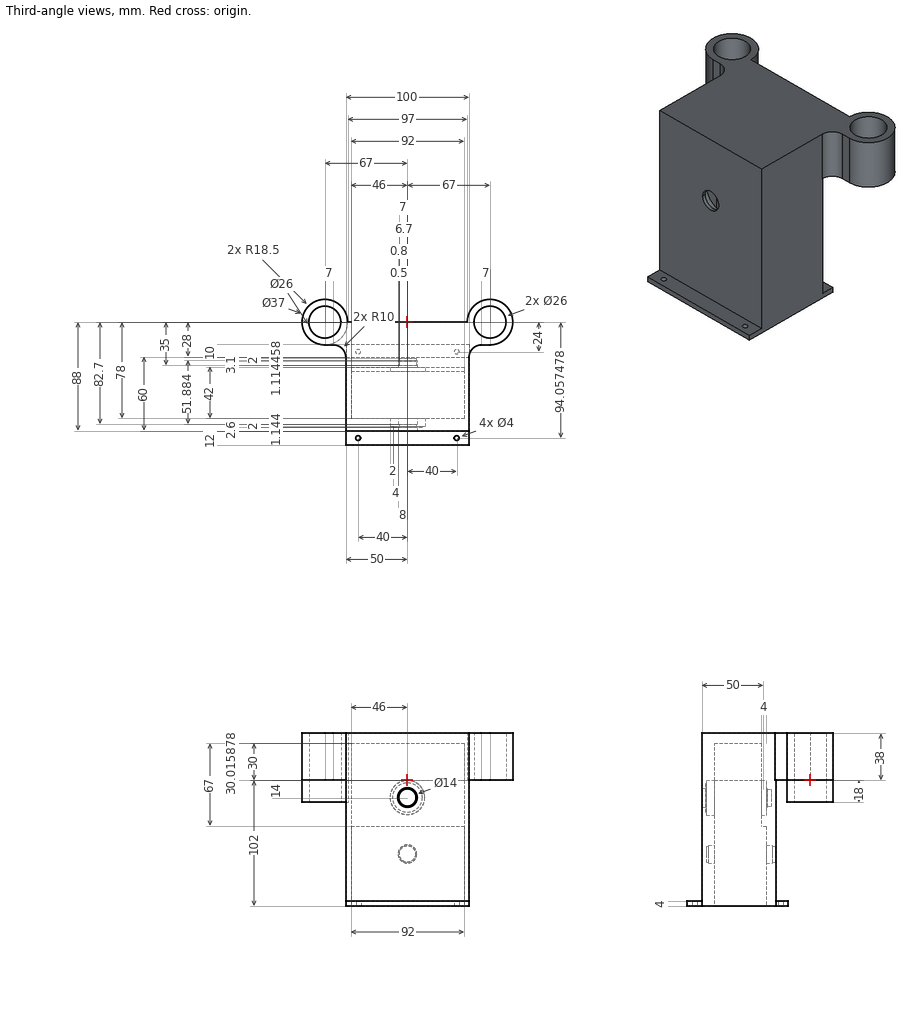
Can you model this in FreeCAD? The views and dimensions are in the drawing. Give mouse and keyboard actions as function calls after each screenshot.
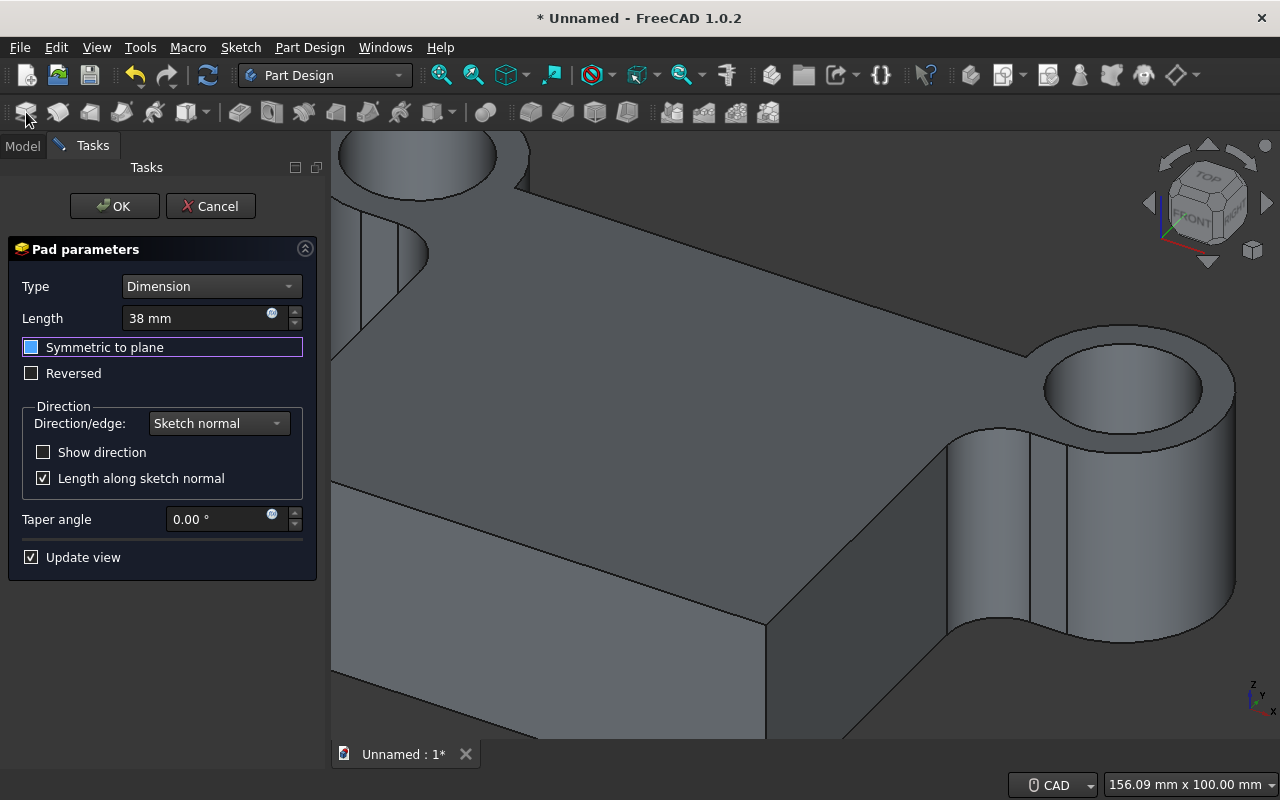
click(115, 206)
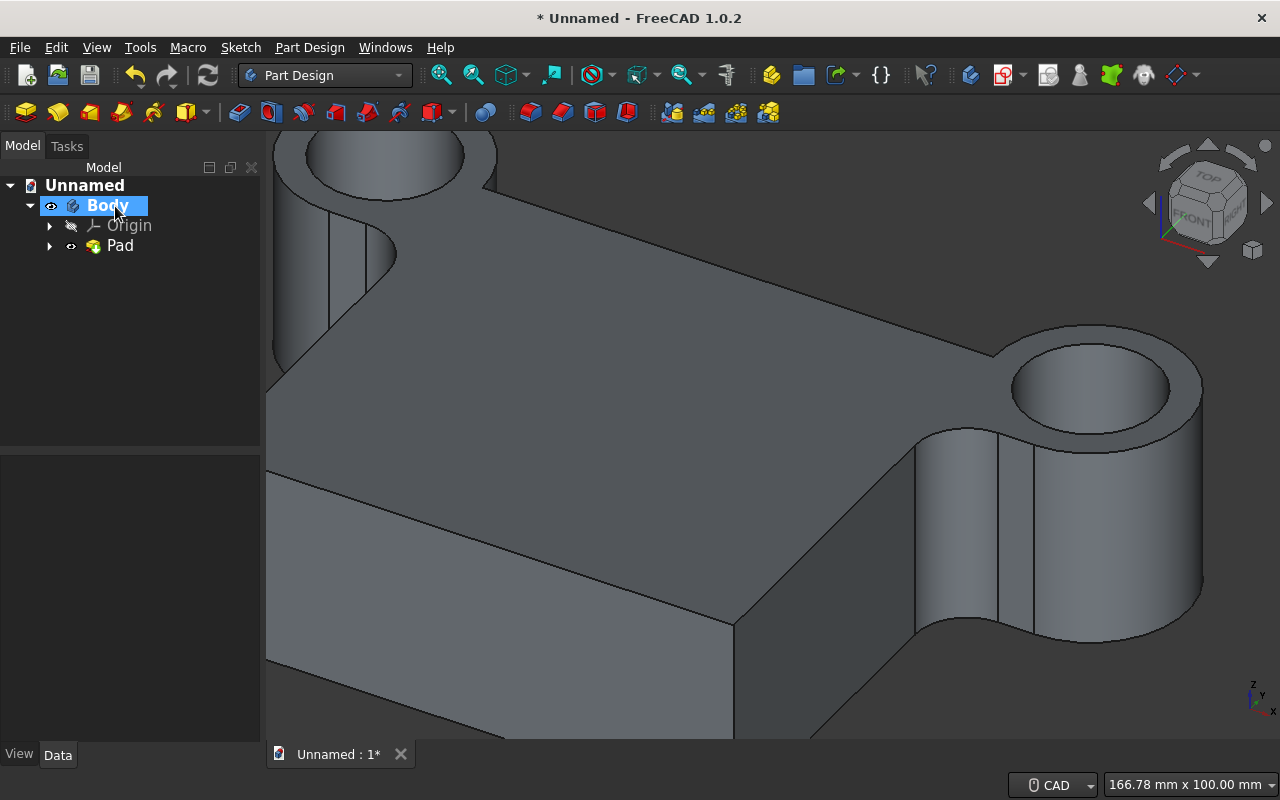
key(v)
key(f)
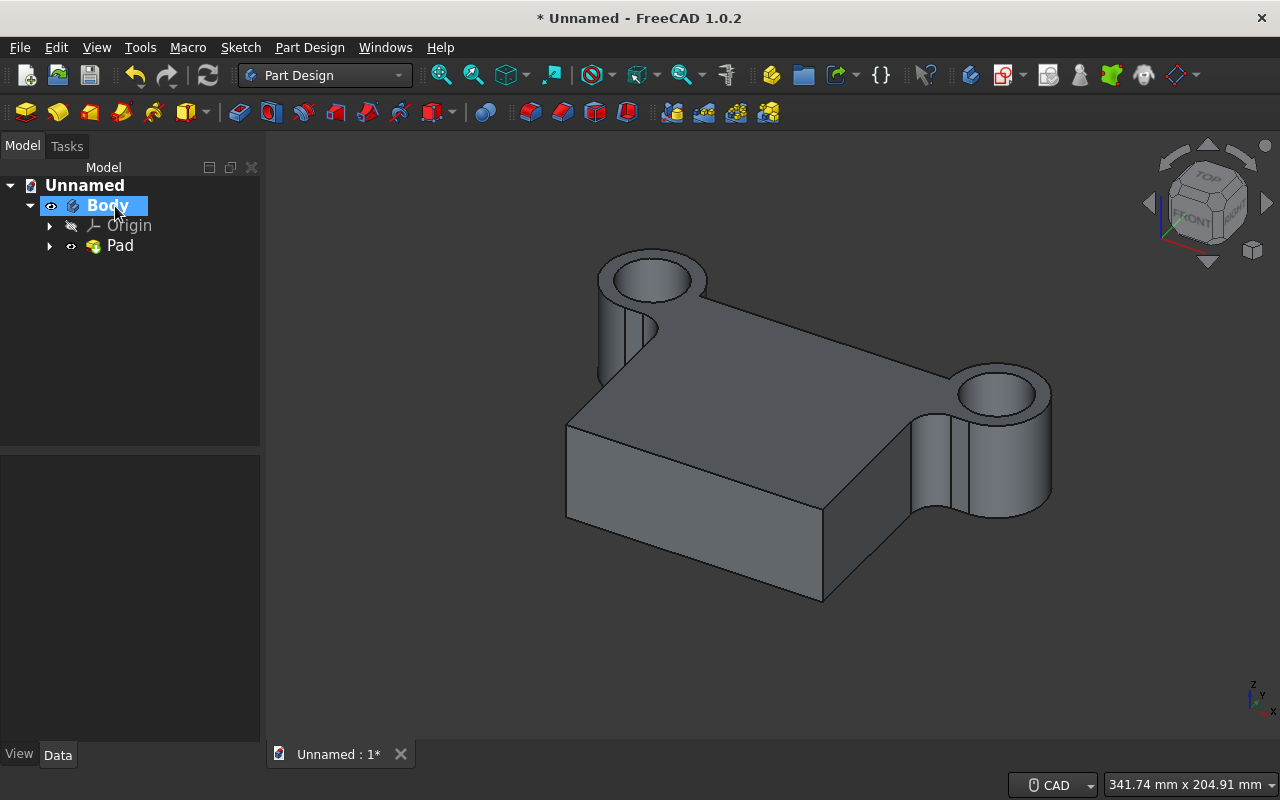
key(5)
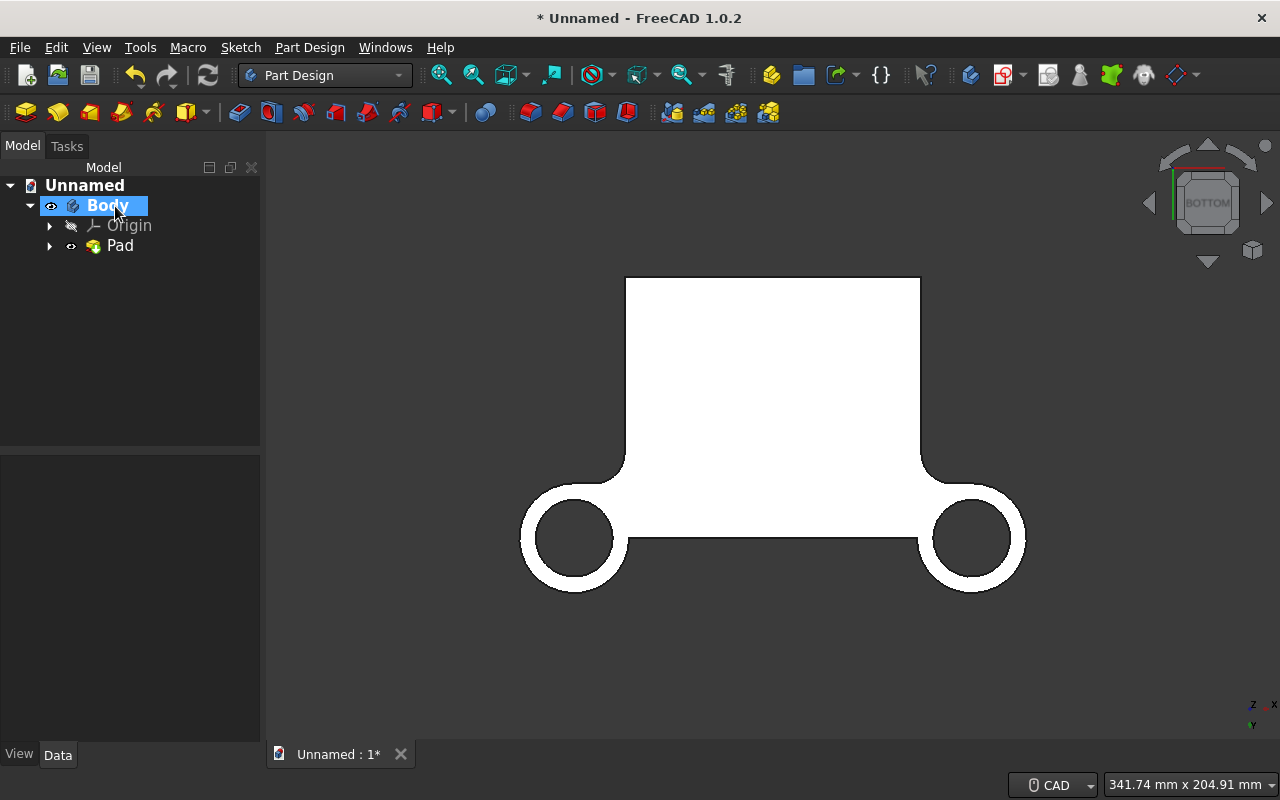
click(773, 389)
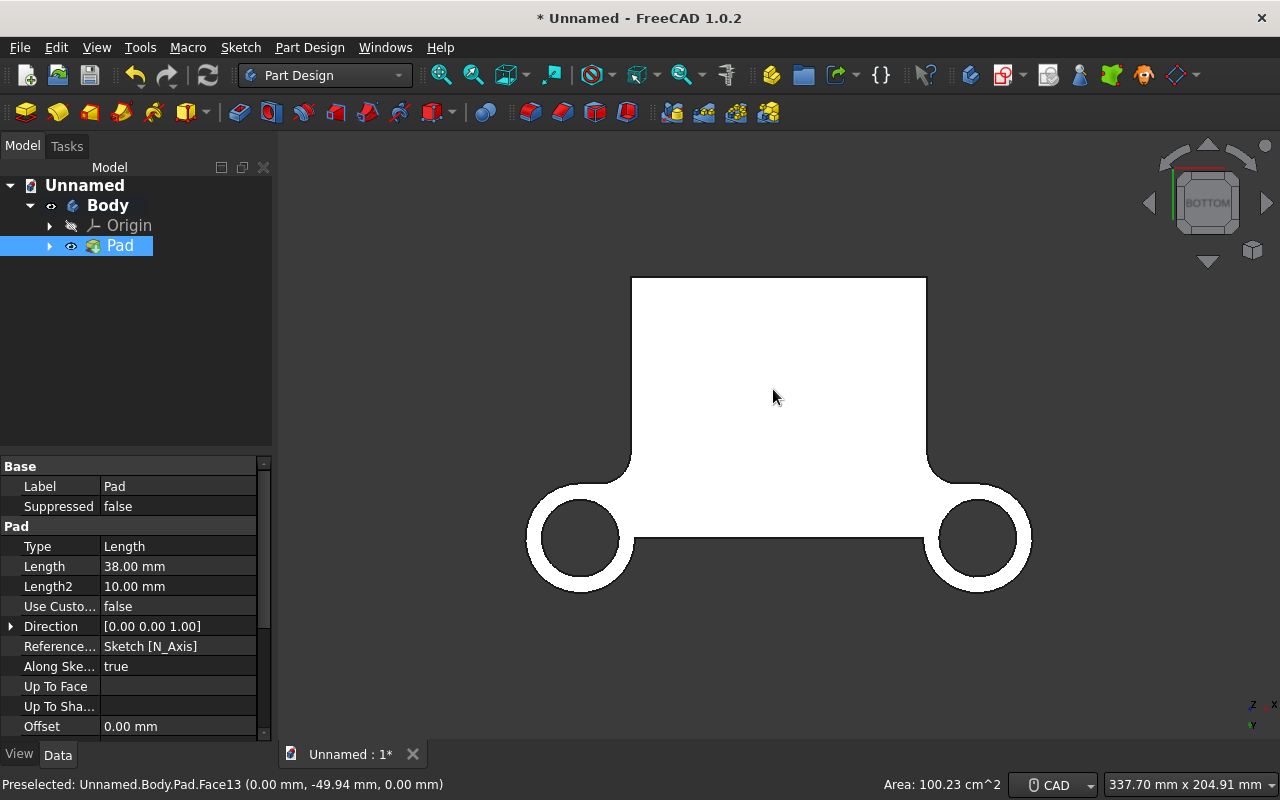
click(1004, 76)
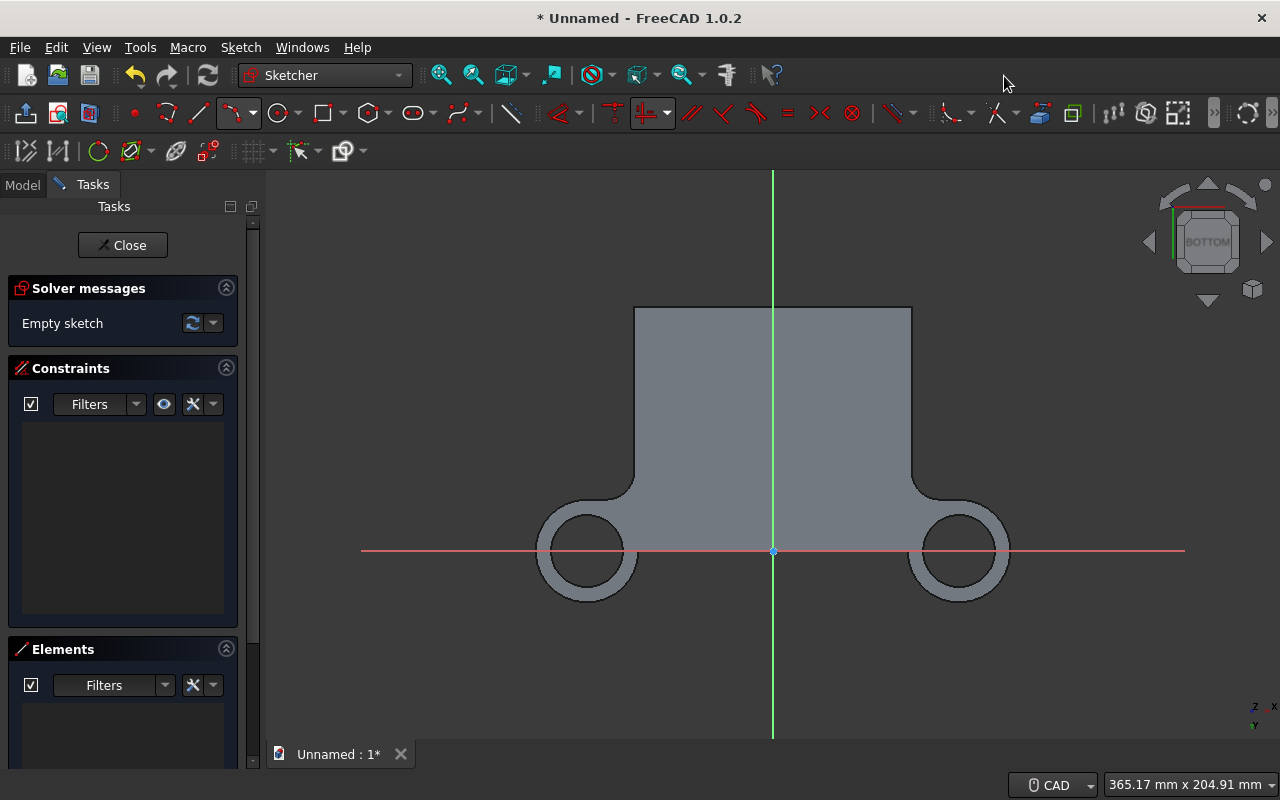
scroll(912, 377, up, 2)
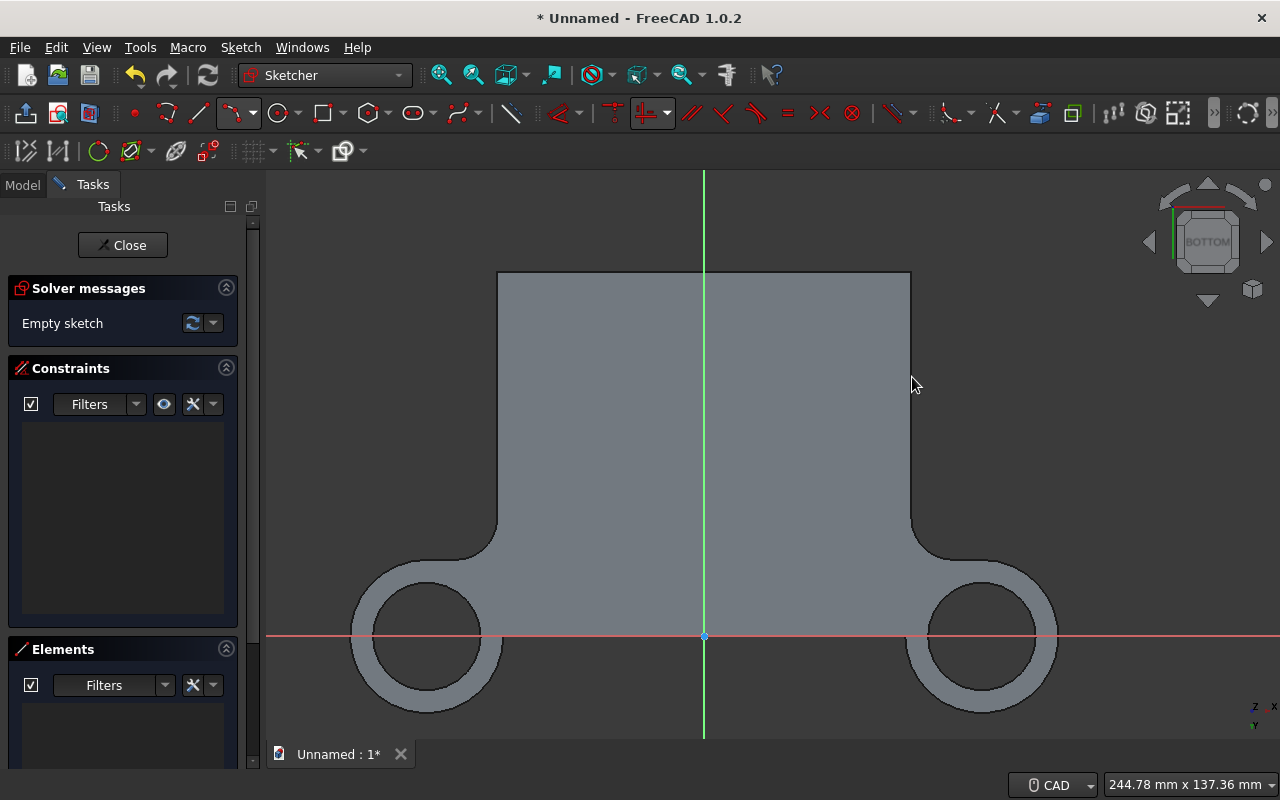
key(g)
key(r)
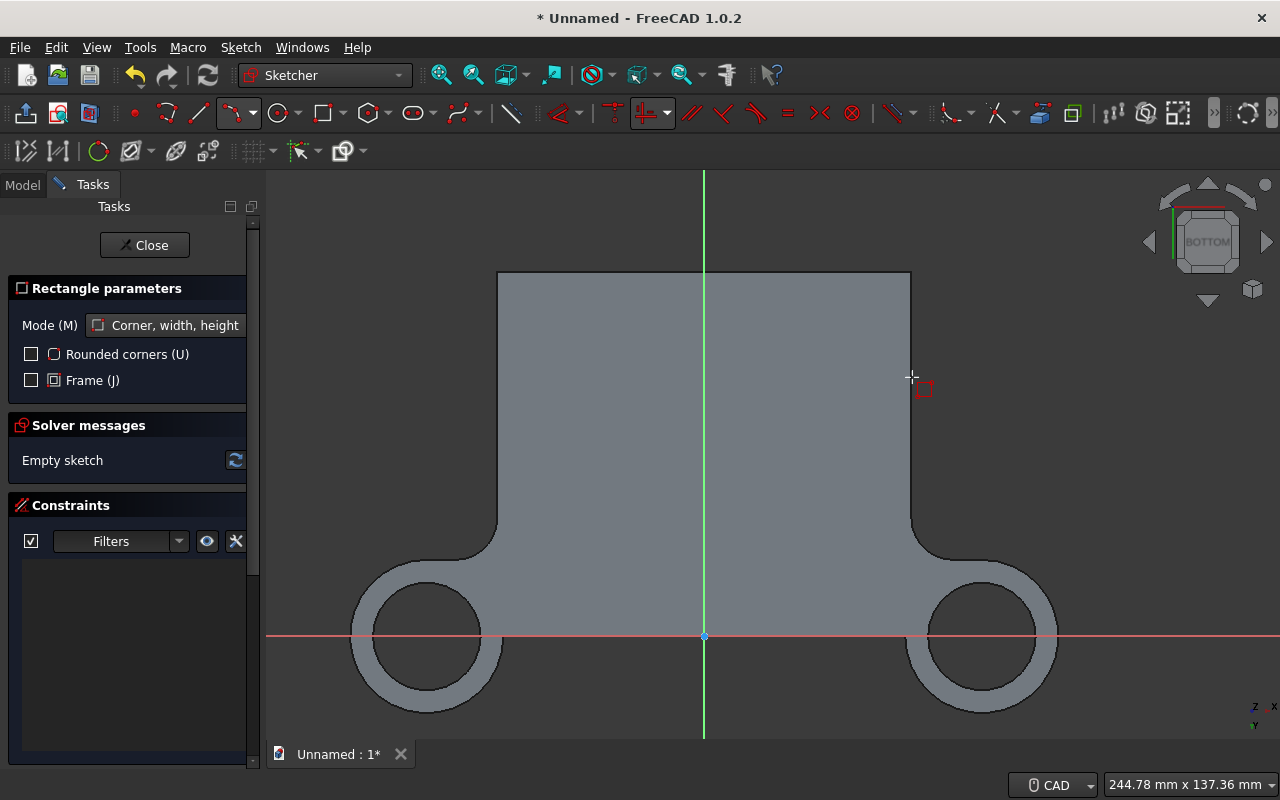
click(497, 272)
click(911, 520)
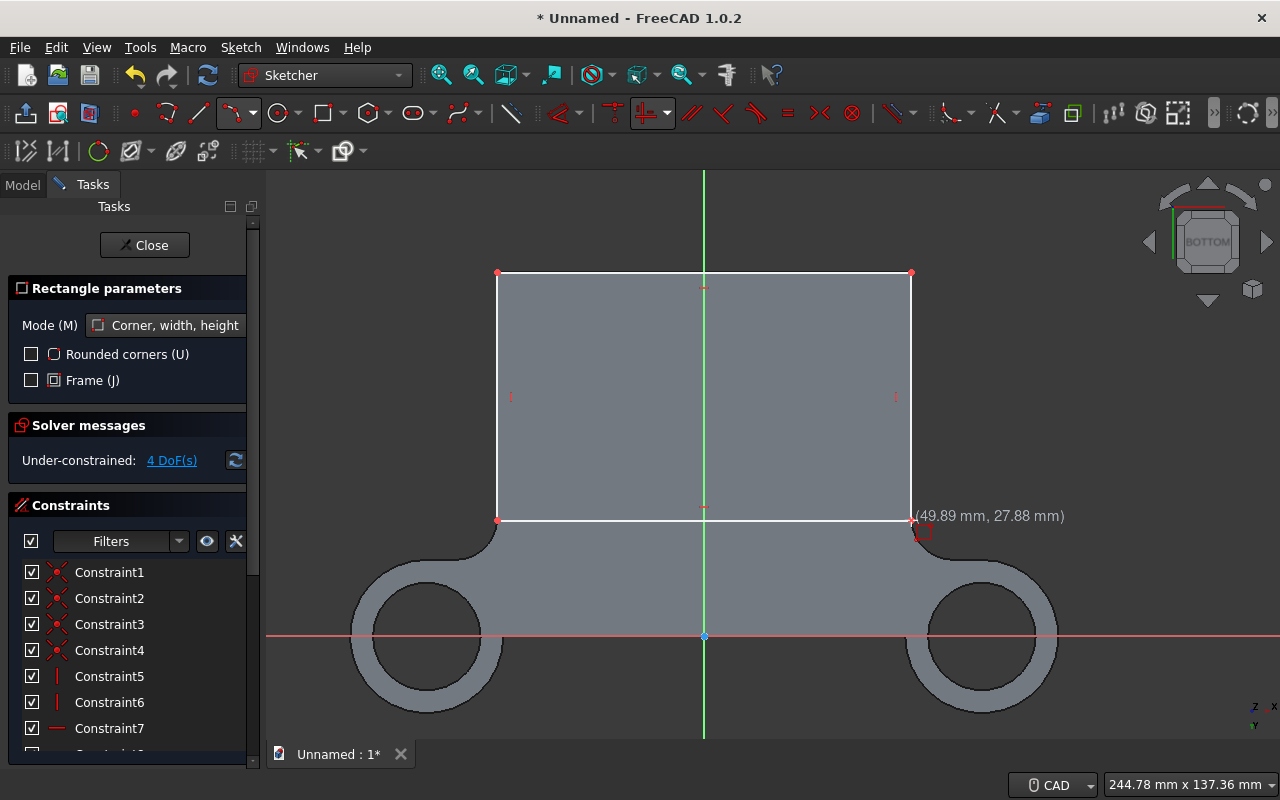
click(514, 313)
click(895, 487)
key(Escape)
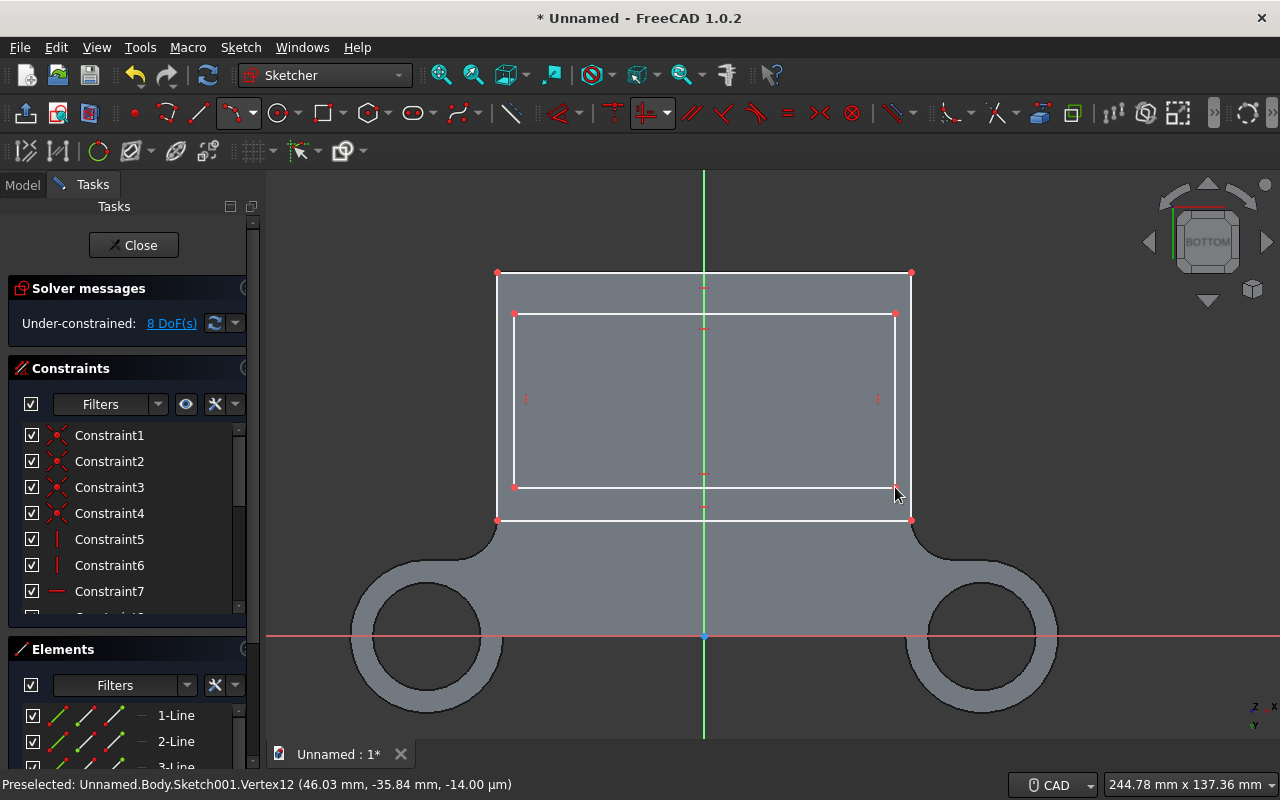
key(d)